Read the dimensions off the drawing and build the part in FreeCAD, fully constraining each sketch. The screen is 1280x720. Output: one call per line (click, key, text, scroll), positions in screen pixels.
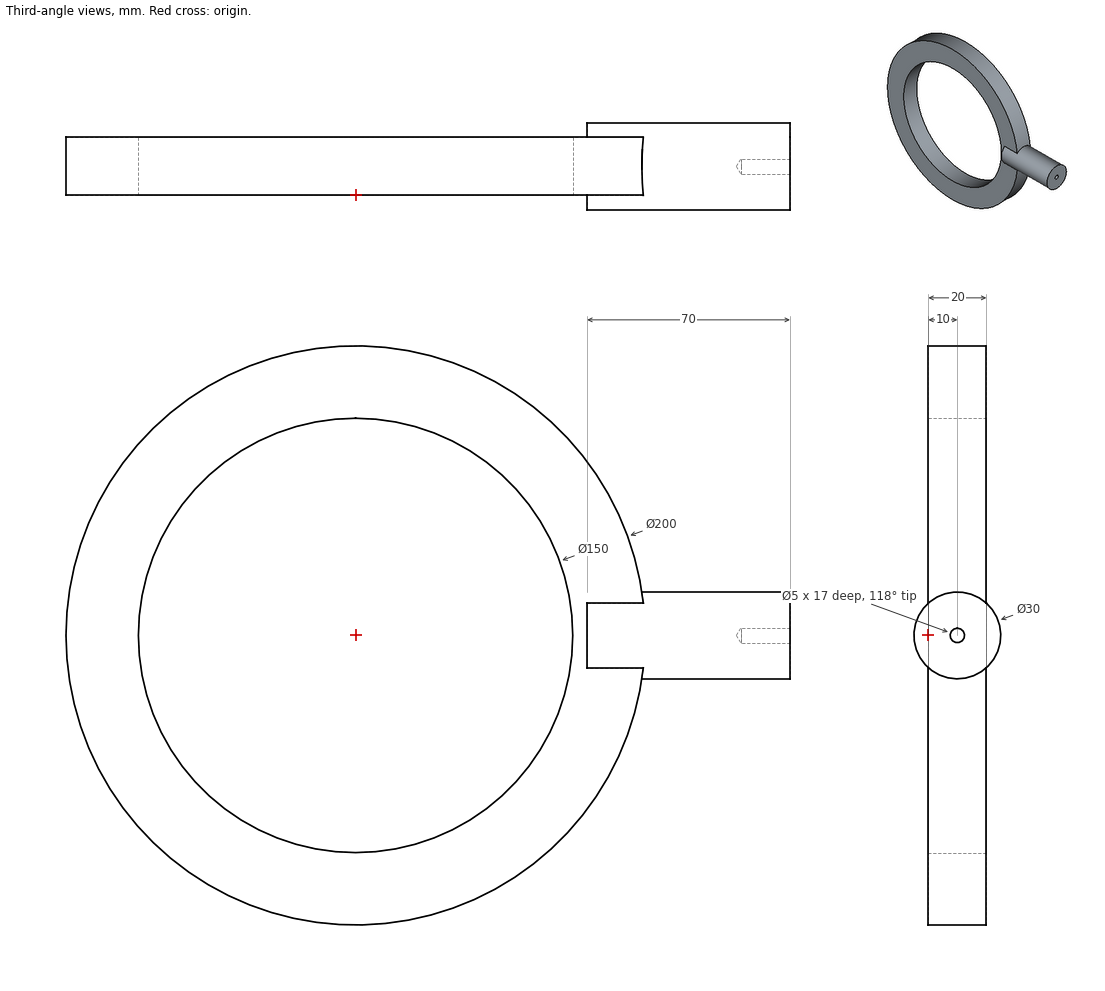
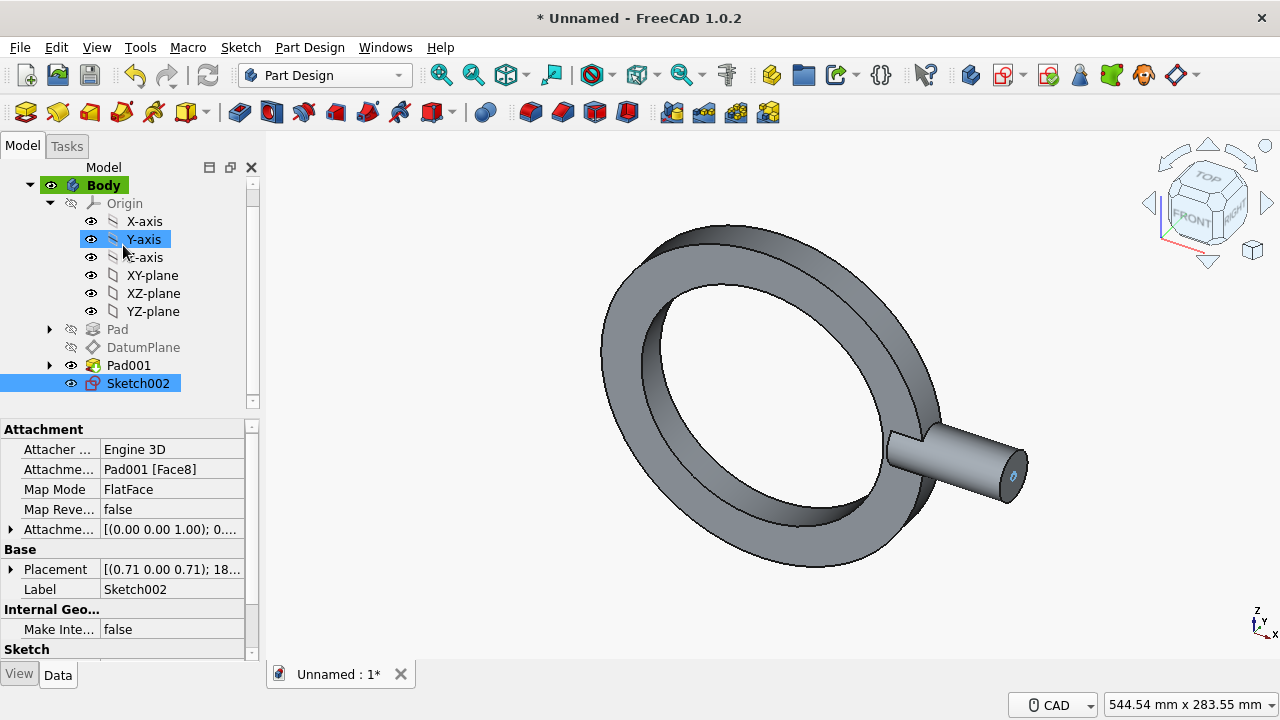
click(272, 112)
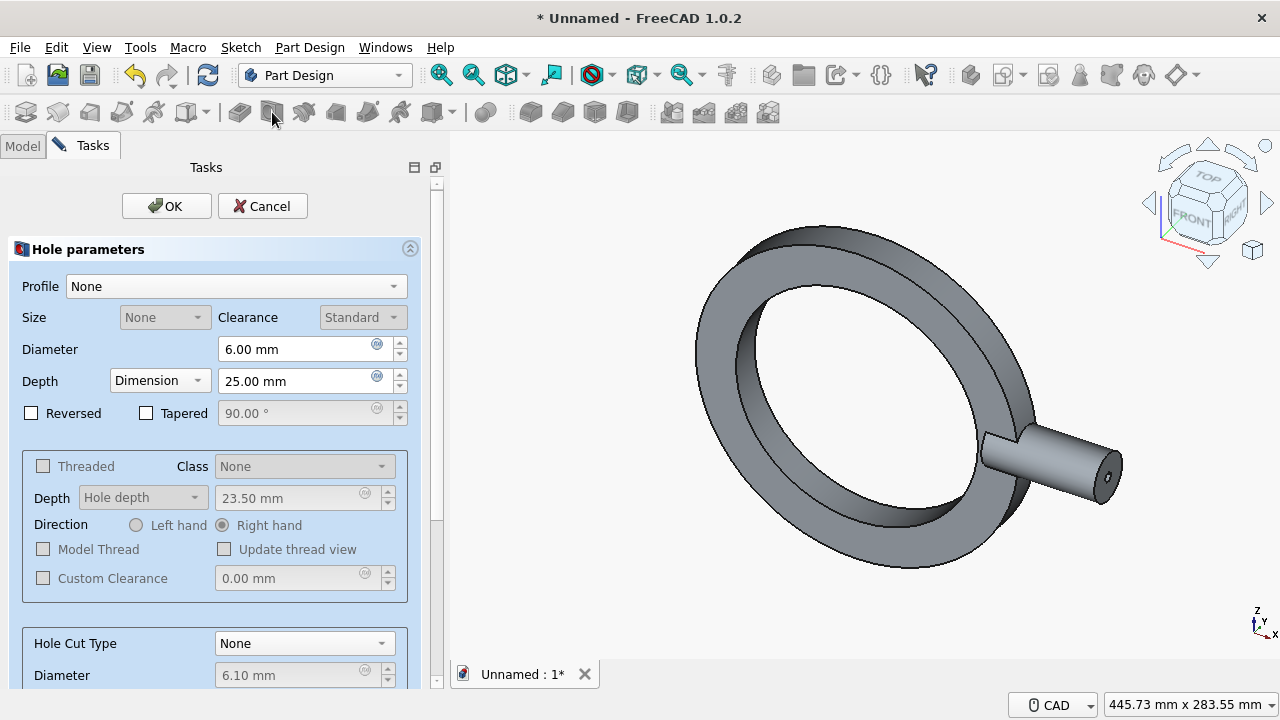
triple_click(305, 349)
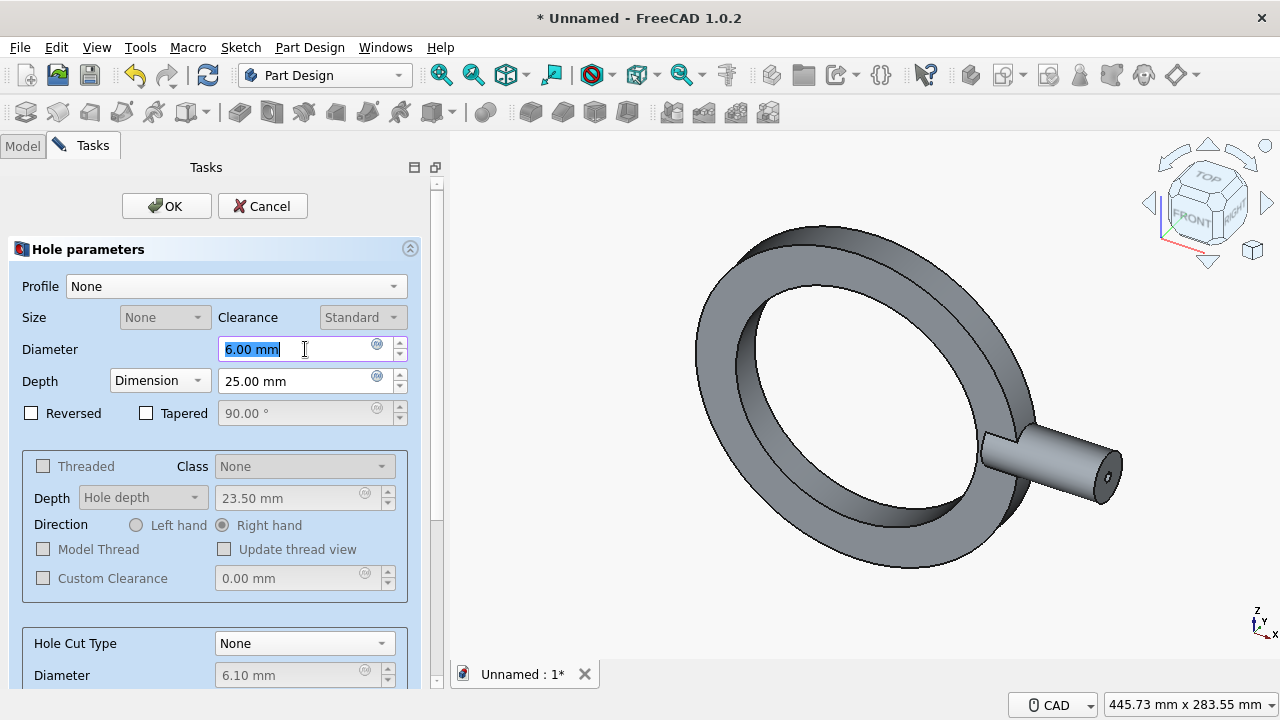
text(5)
key(Tab)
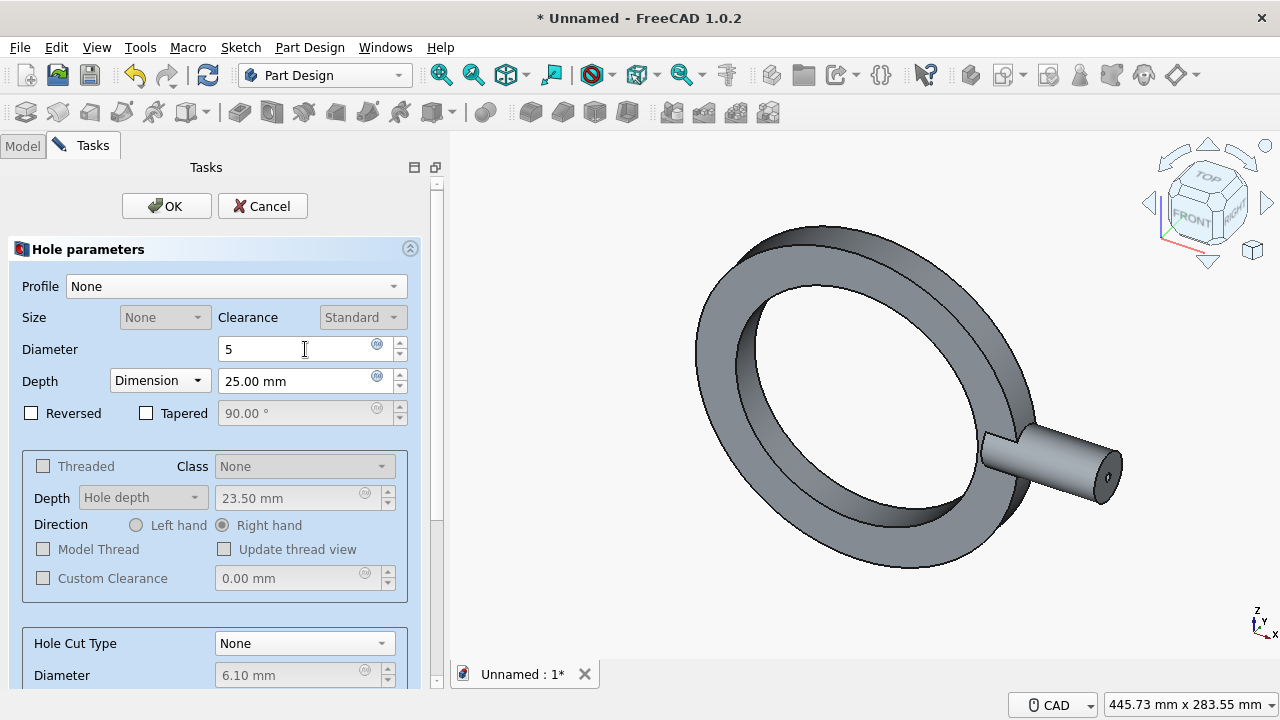
triple_click(305, 381)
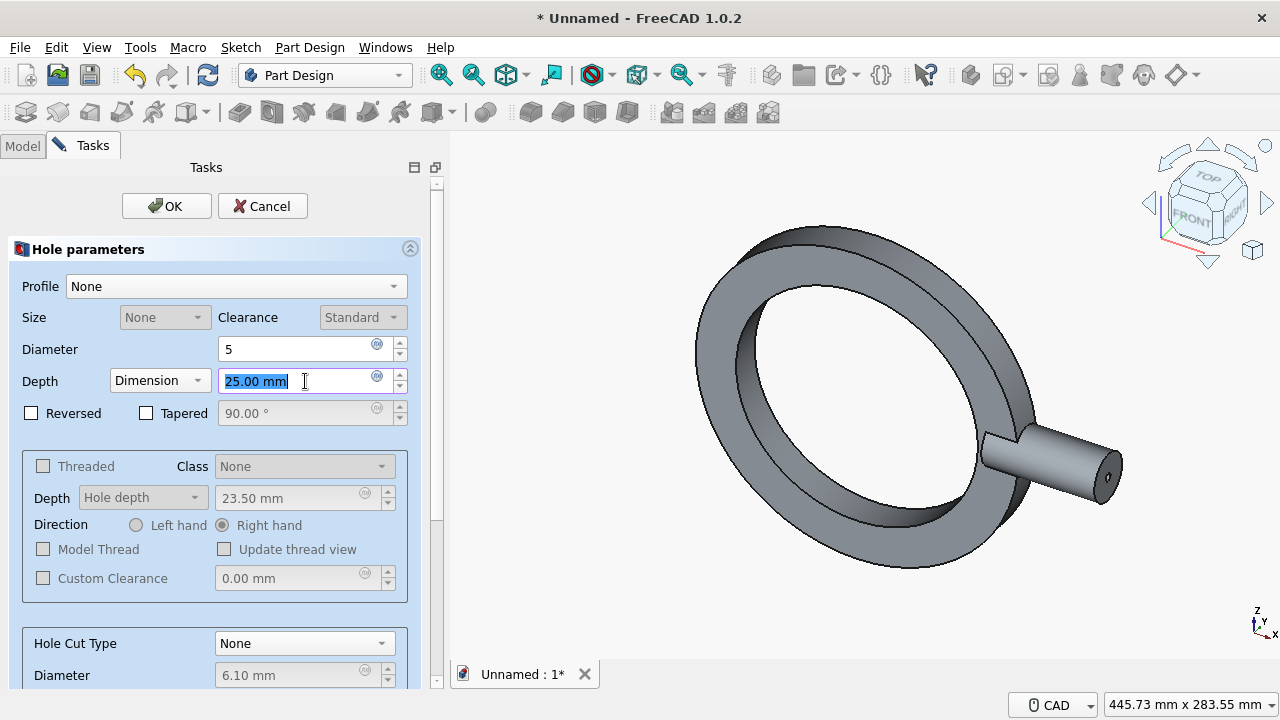
text(17)
key(Tab)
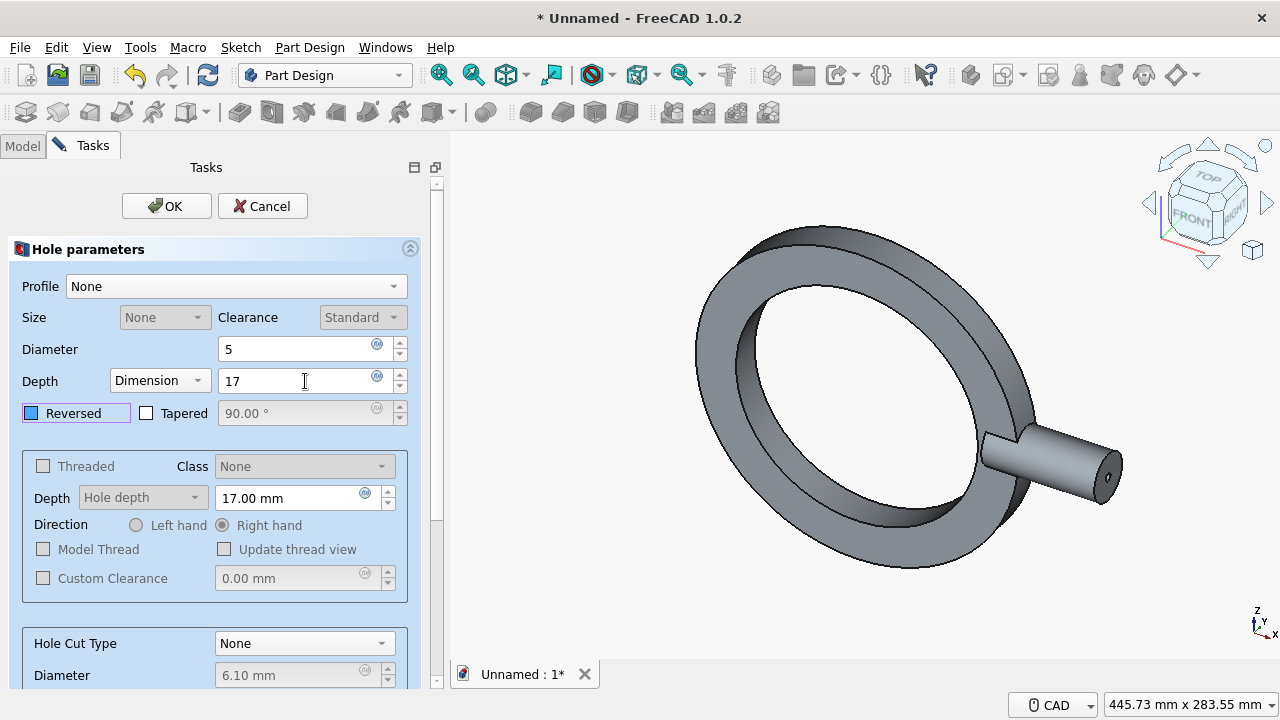
click(167, 206)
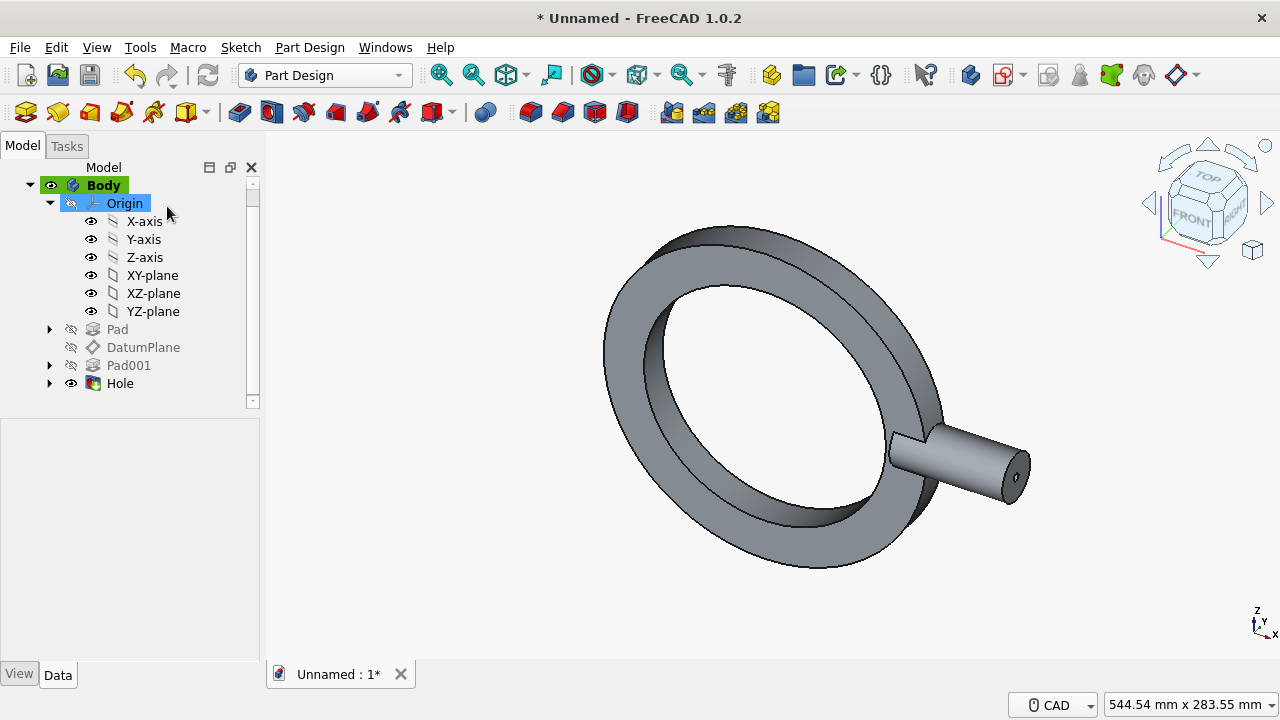
key(0)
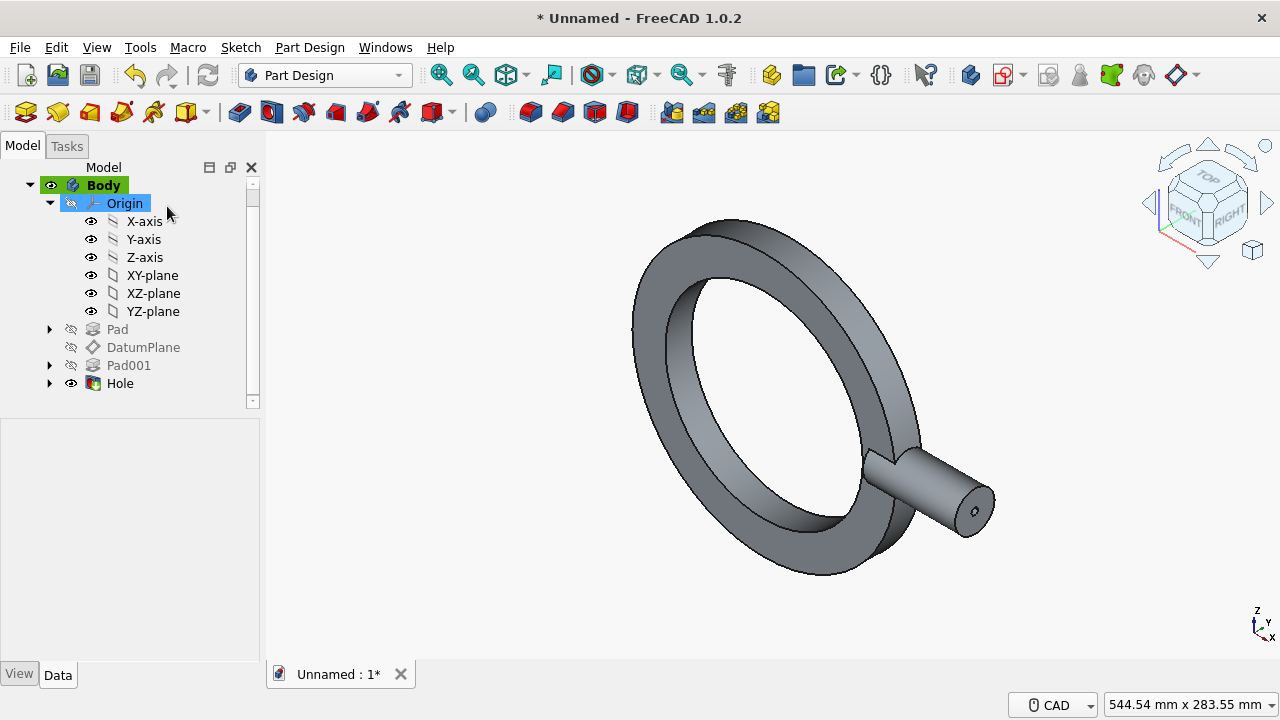
key(v)
key(f)